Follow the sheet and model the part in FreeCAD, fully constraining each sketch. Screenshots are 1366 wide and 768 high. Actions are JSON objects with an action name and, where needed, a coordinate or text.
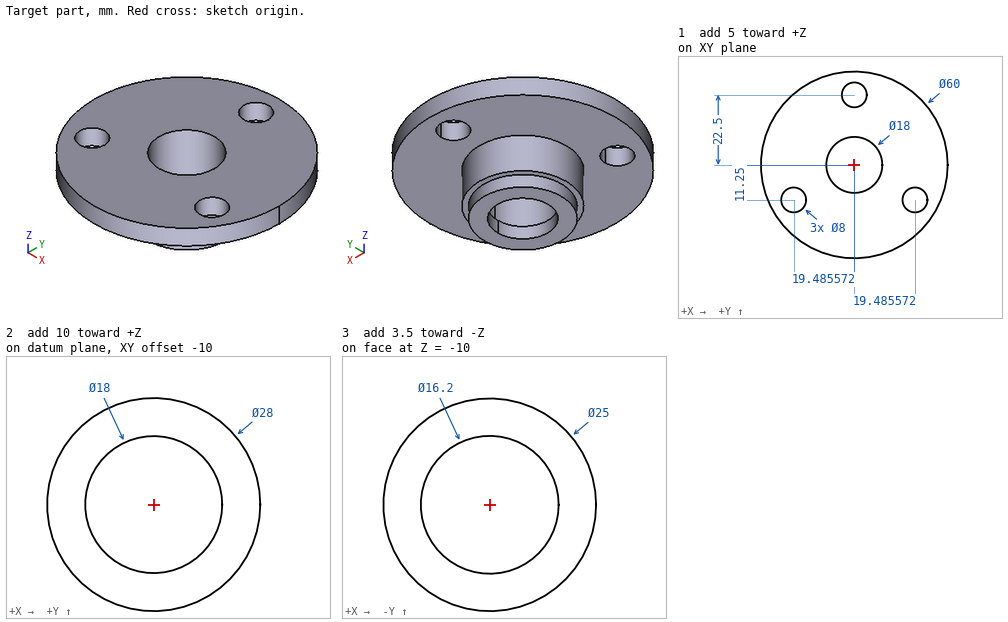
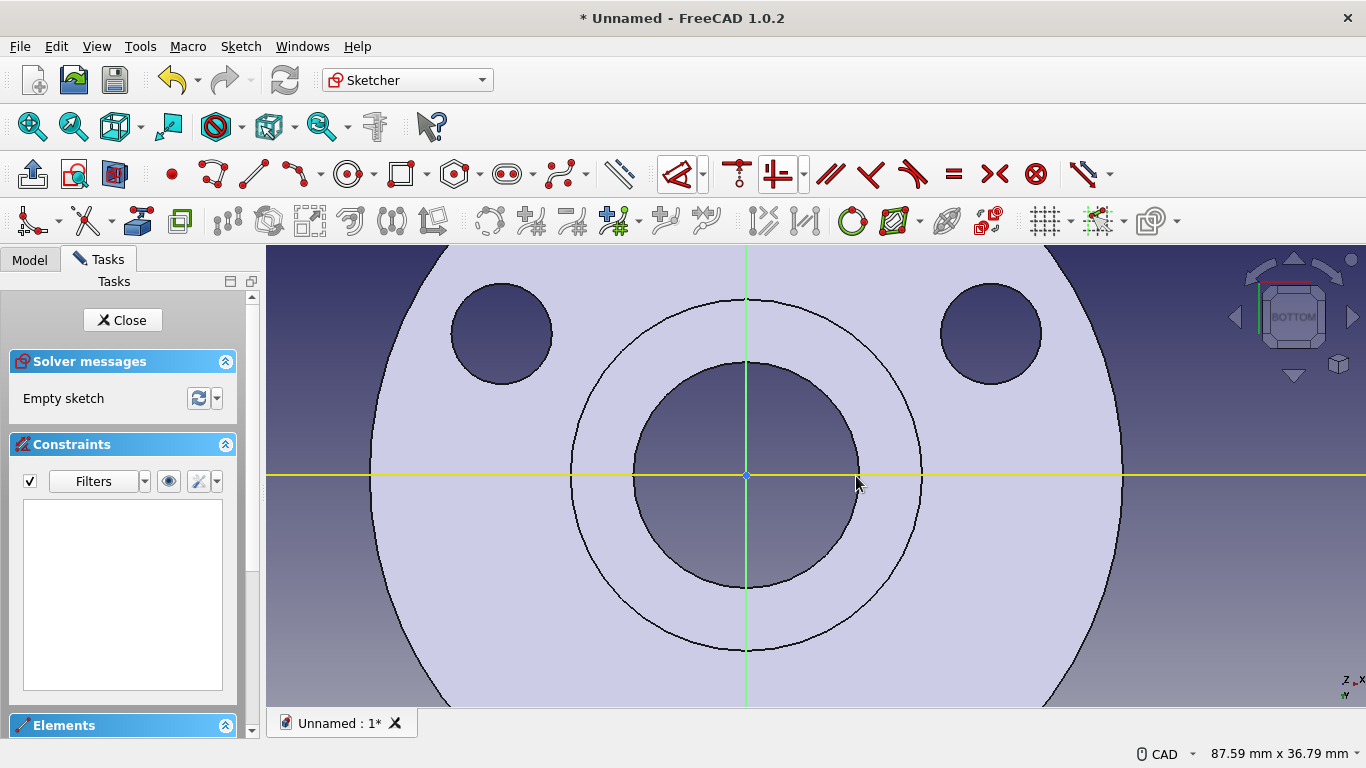
{"action": "key", "text": "g c"}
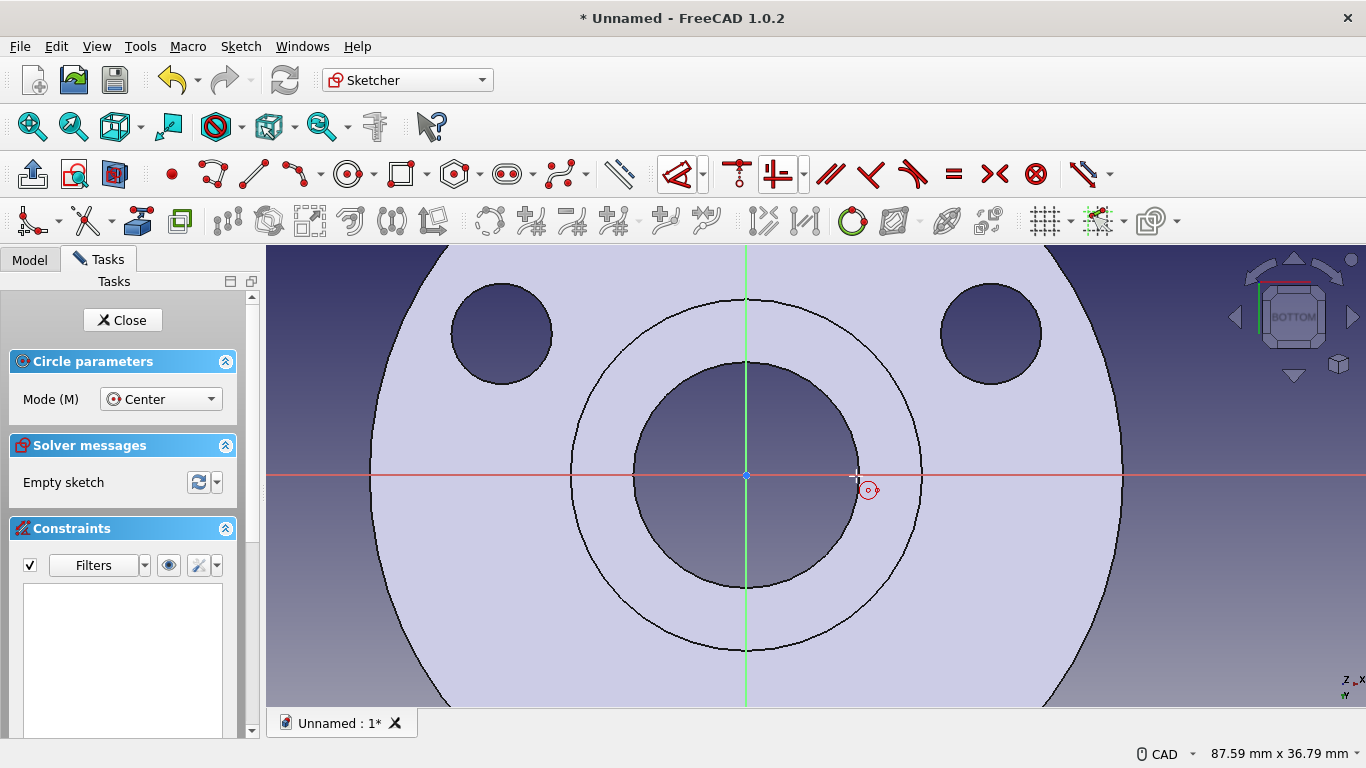
{"action": "left_click", "coordinate": [746, 475]}
{"action": "mouse_move", "coordinate": [857, 364]}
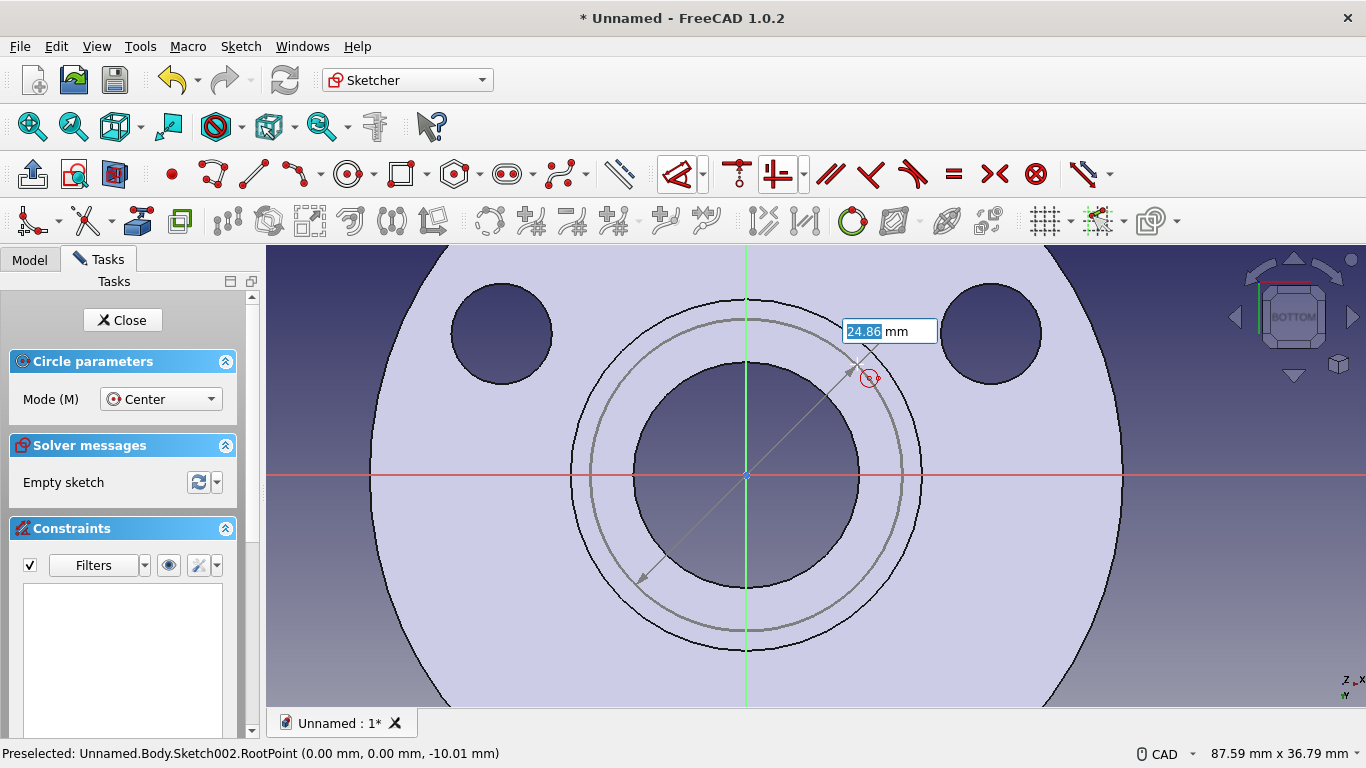
{"action": "type", "text": "25"}
{"action": "key", "text": "Return"}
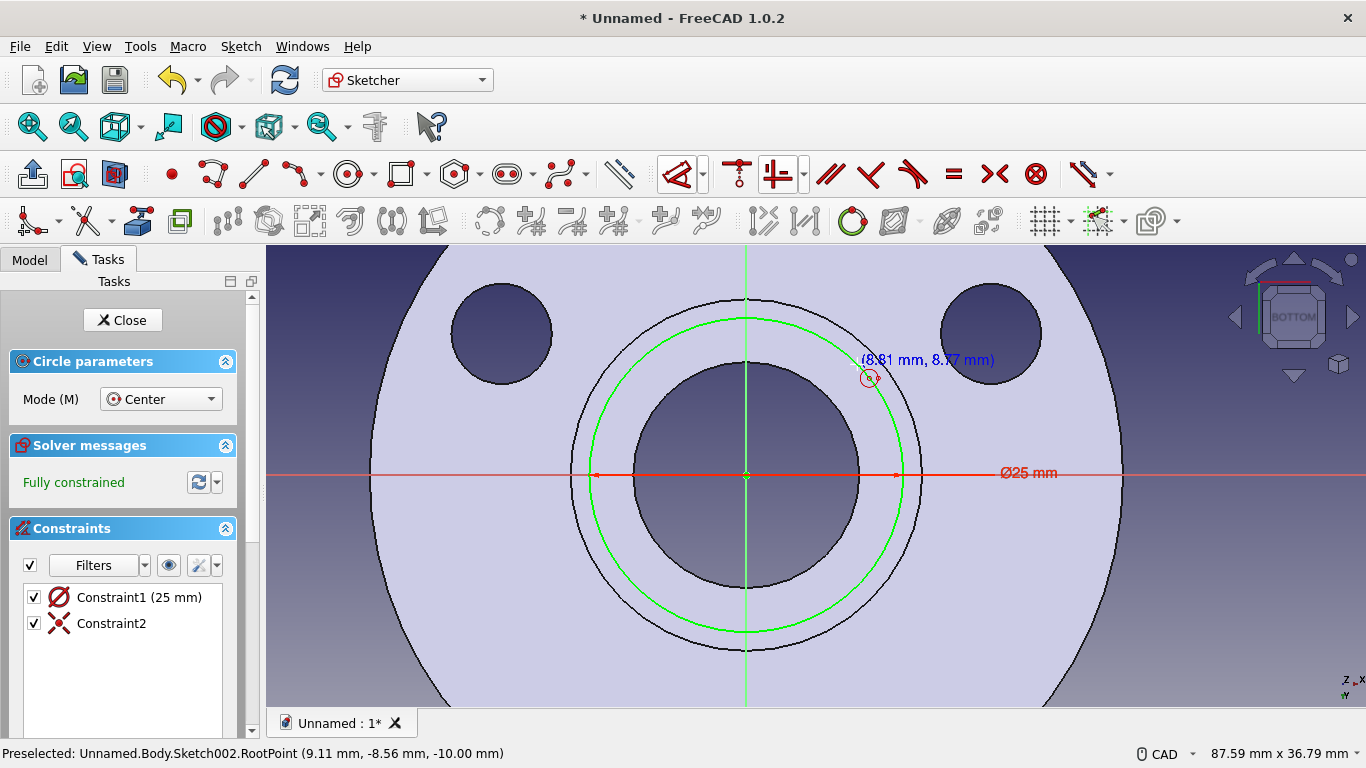
{"action": "left_click", "coordinate": [746, 475]}
{"action": "mouse_move", "coordinate": [818, 403]}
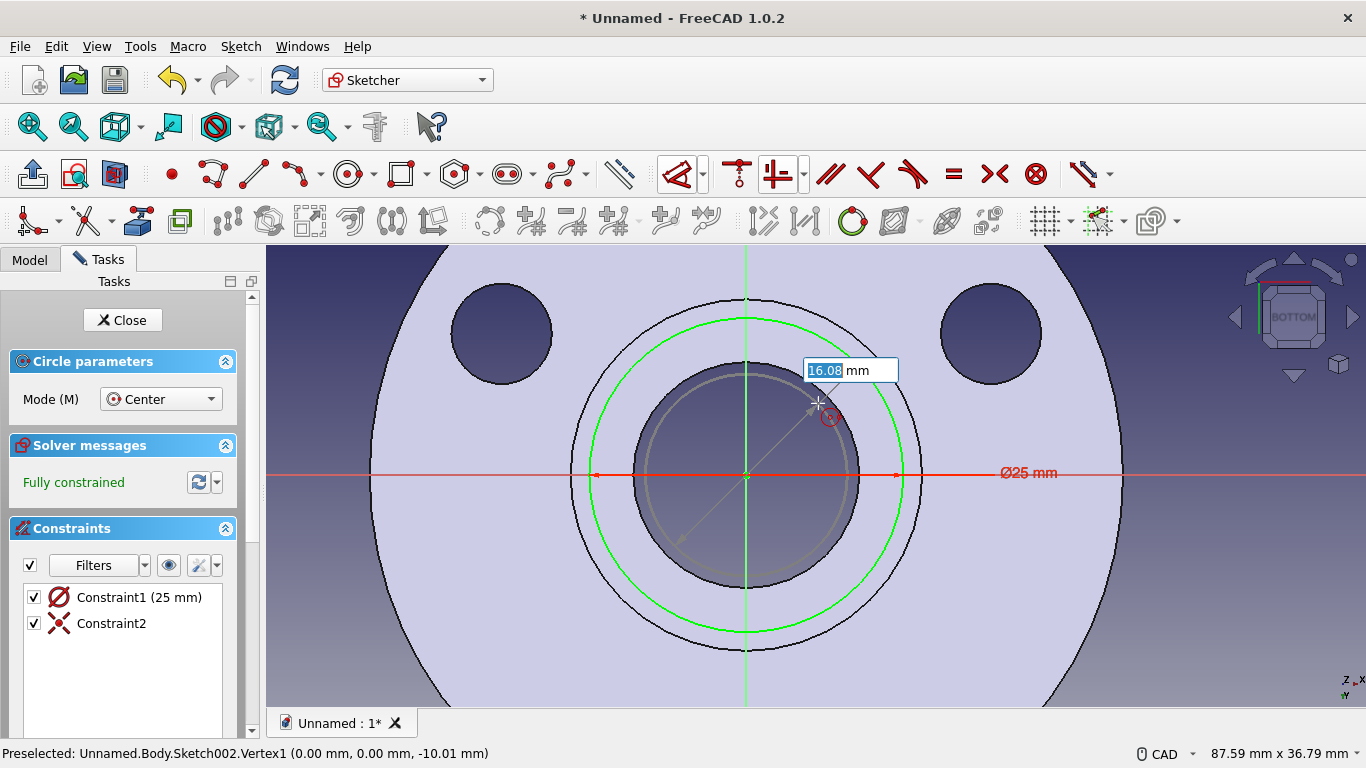
{"action": "type", "text": "16.2"}
{"action": "key", "text": "Return"}
{"action": "key", "text": "Escape"}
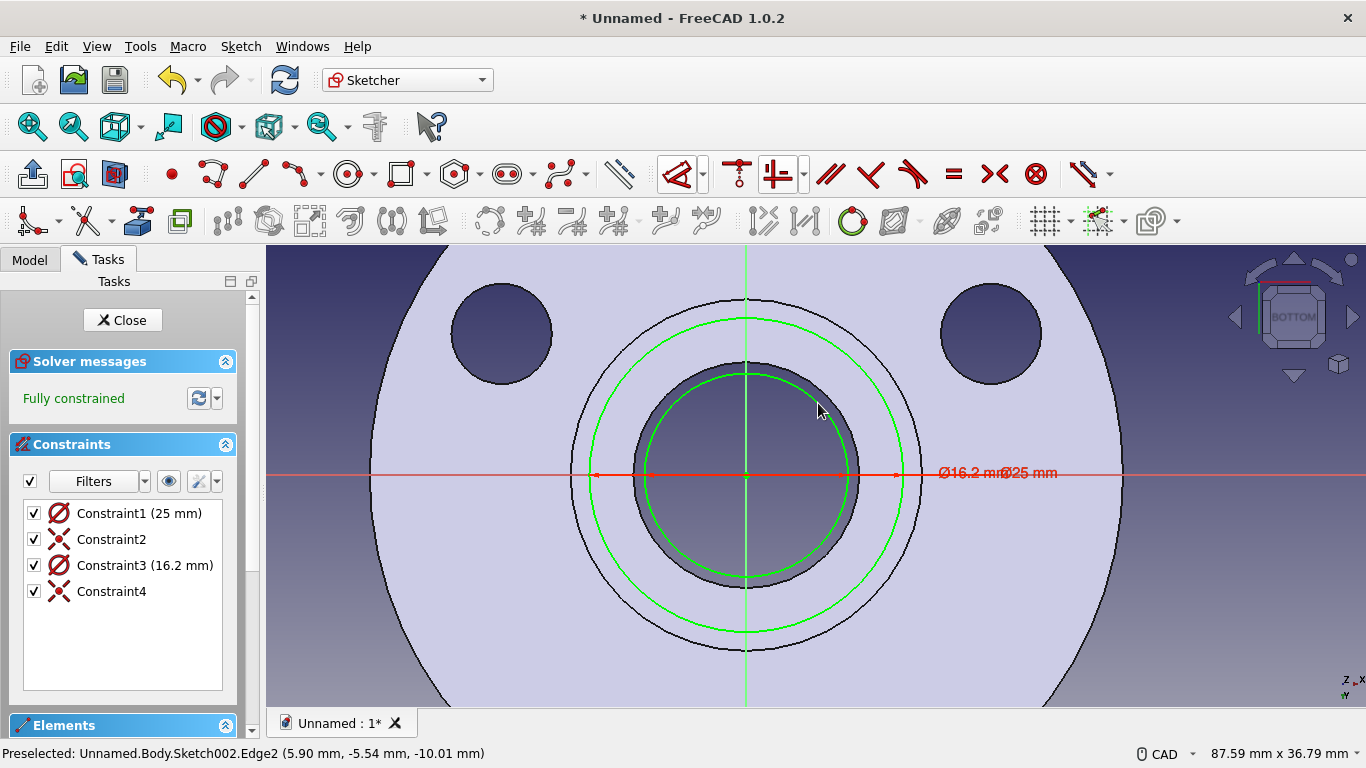
{"action": "left_click", "coordinate": [123, 320]}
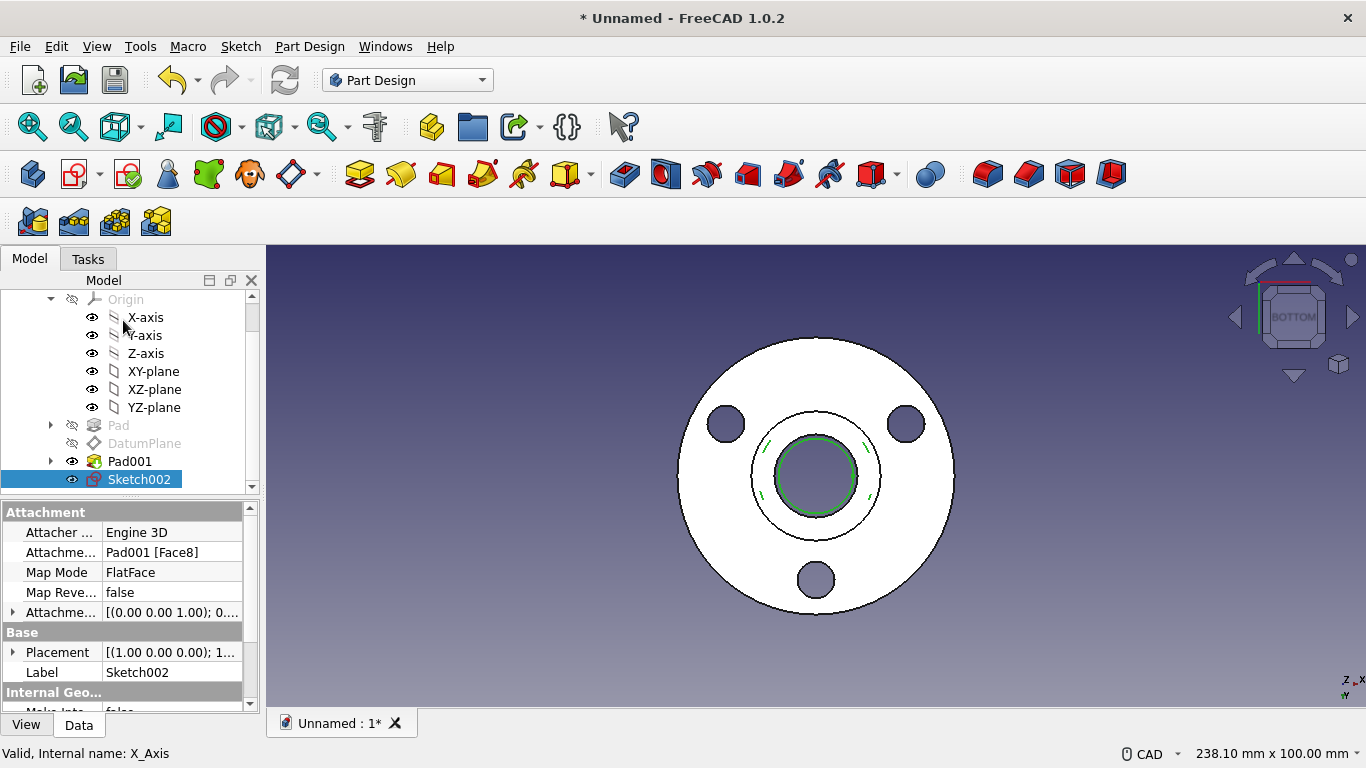
{"action": "left_click", "coordinate": [360, 174]}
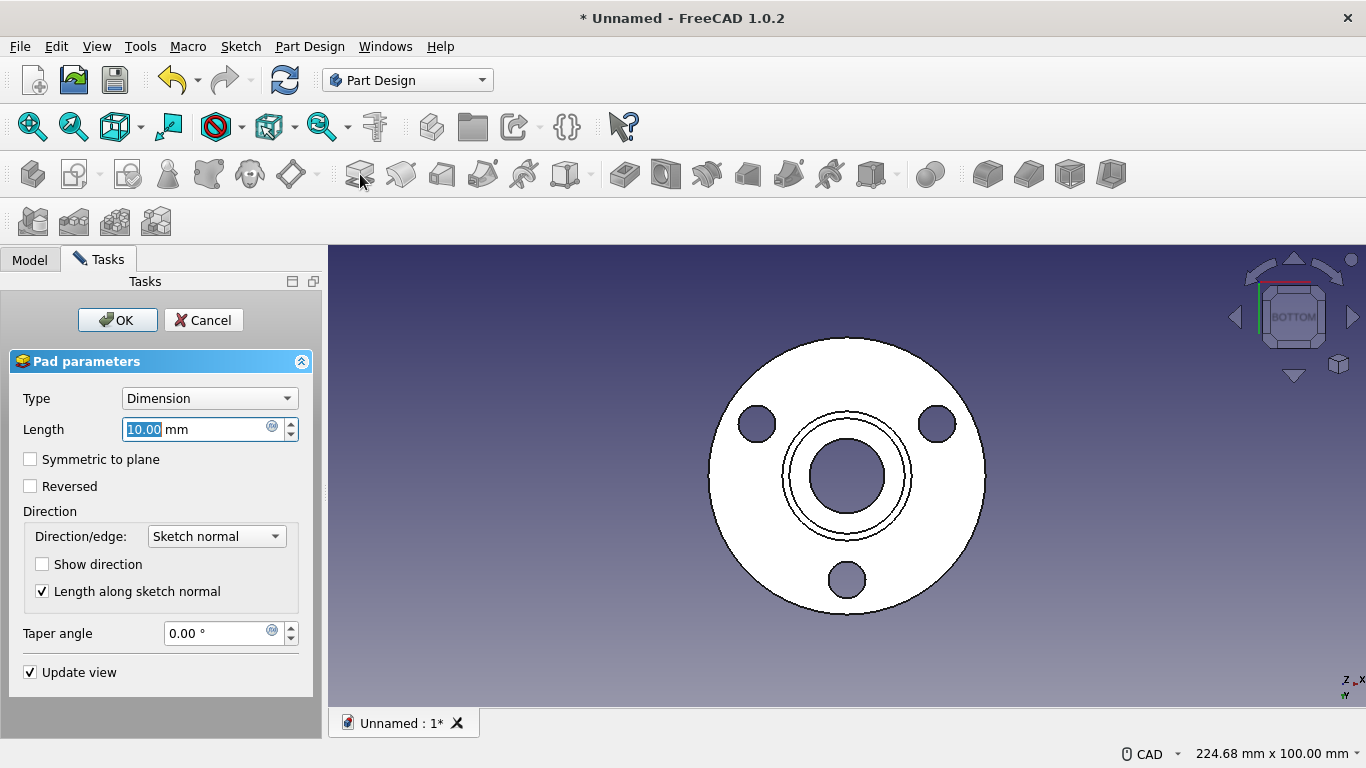
{"action": "type", "text": "3.5"}
{"action": "key", "text": "Tab"}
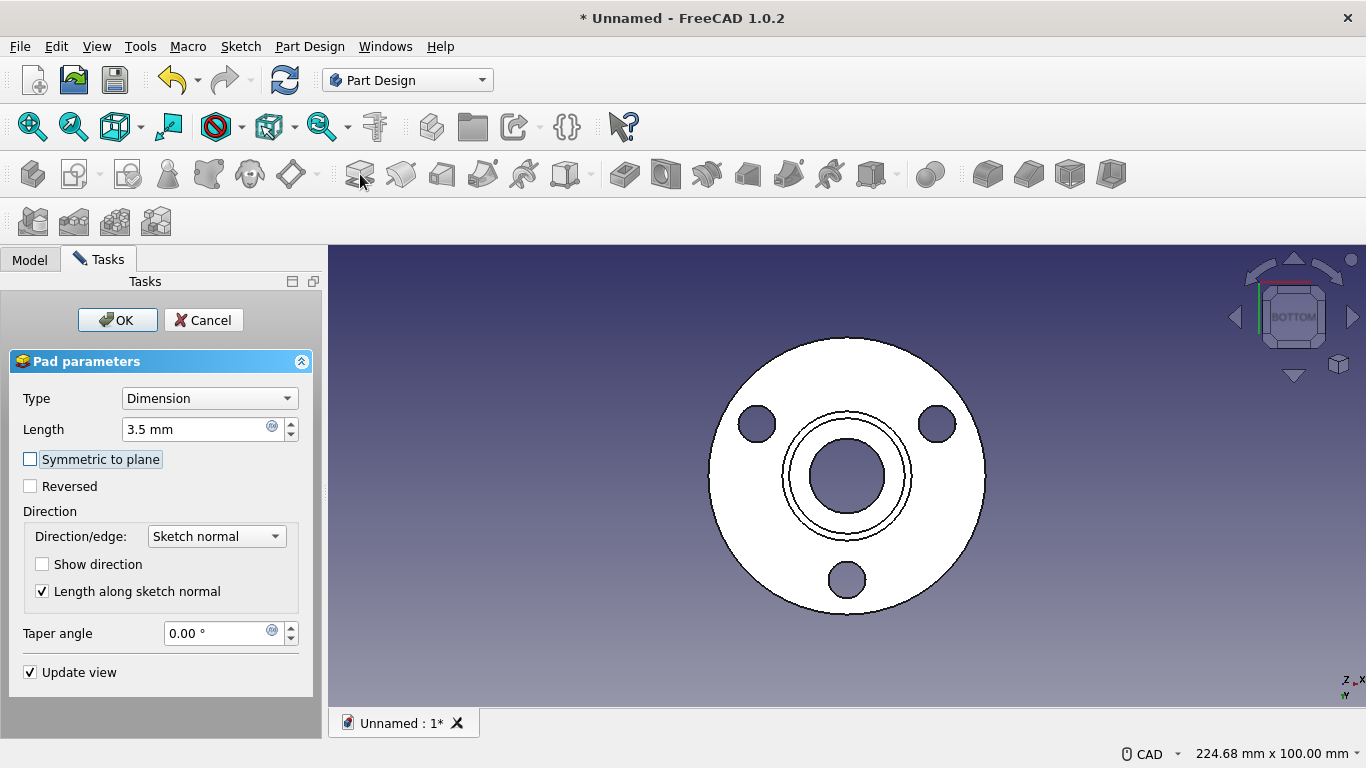
{"action": "left_click", "coordinate": [118, 320]}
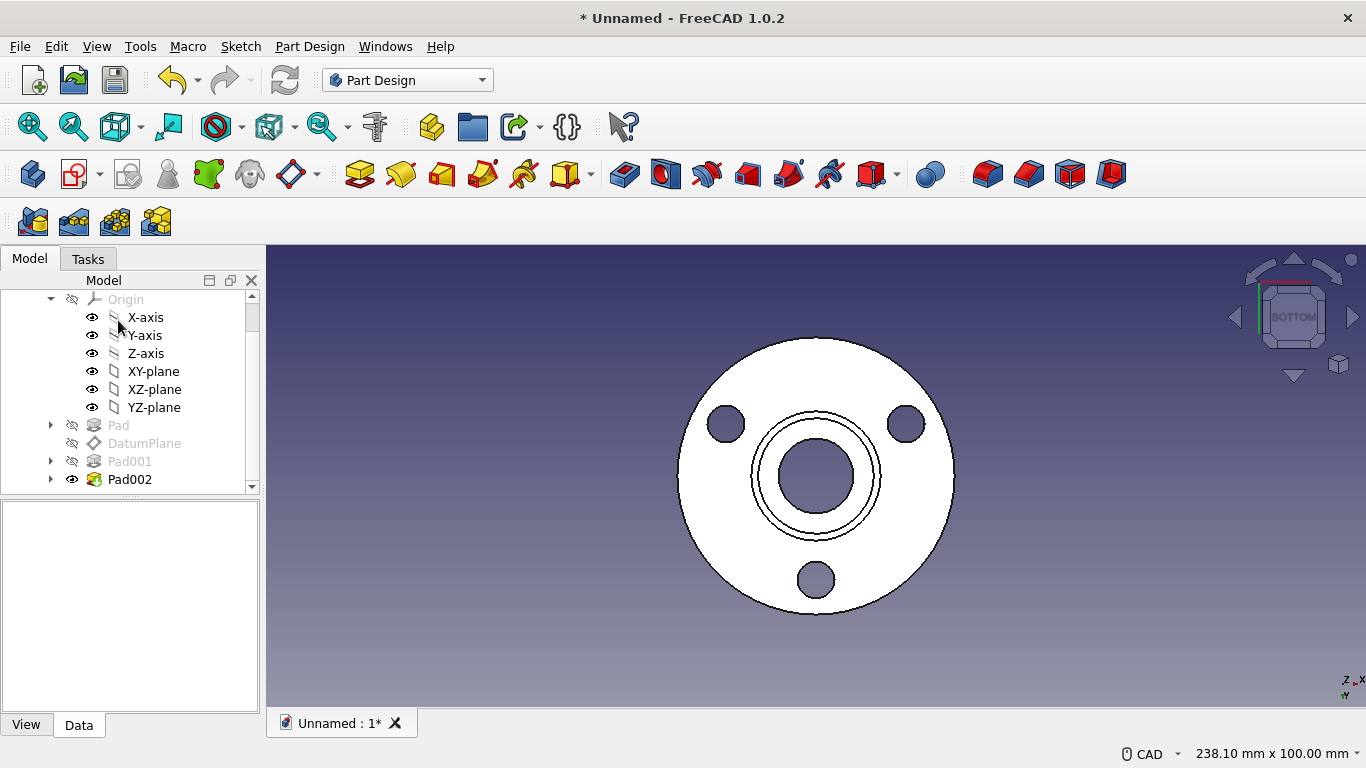
{"action": "key", "text": "0"}